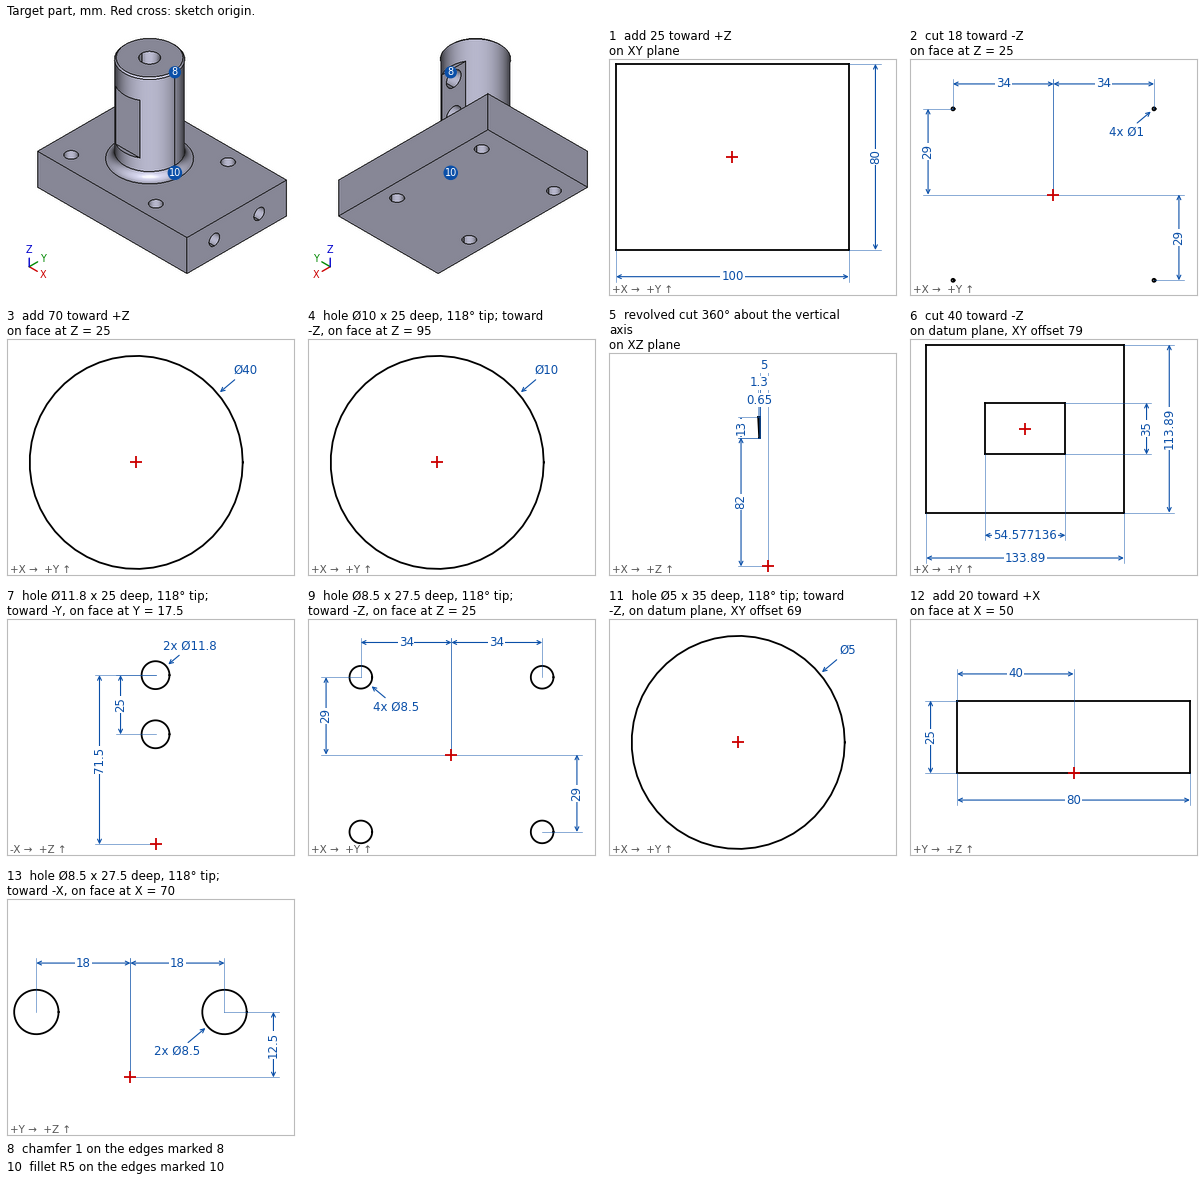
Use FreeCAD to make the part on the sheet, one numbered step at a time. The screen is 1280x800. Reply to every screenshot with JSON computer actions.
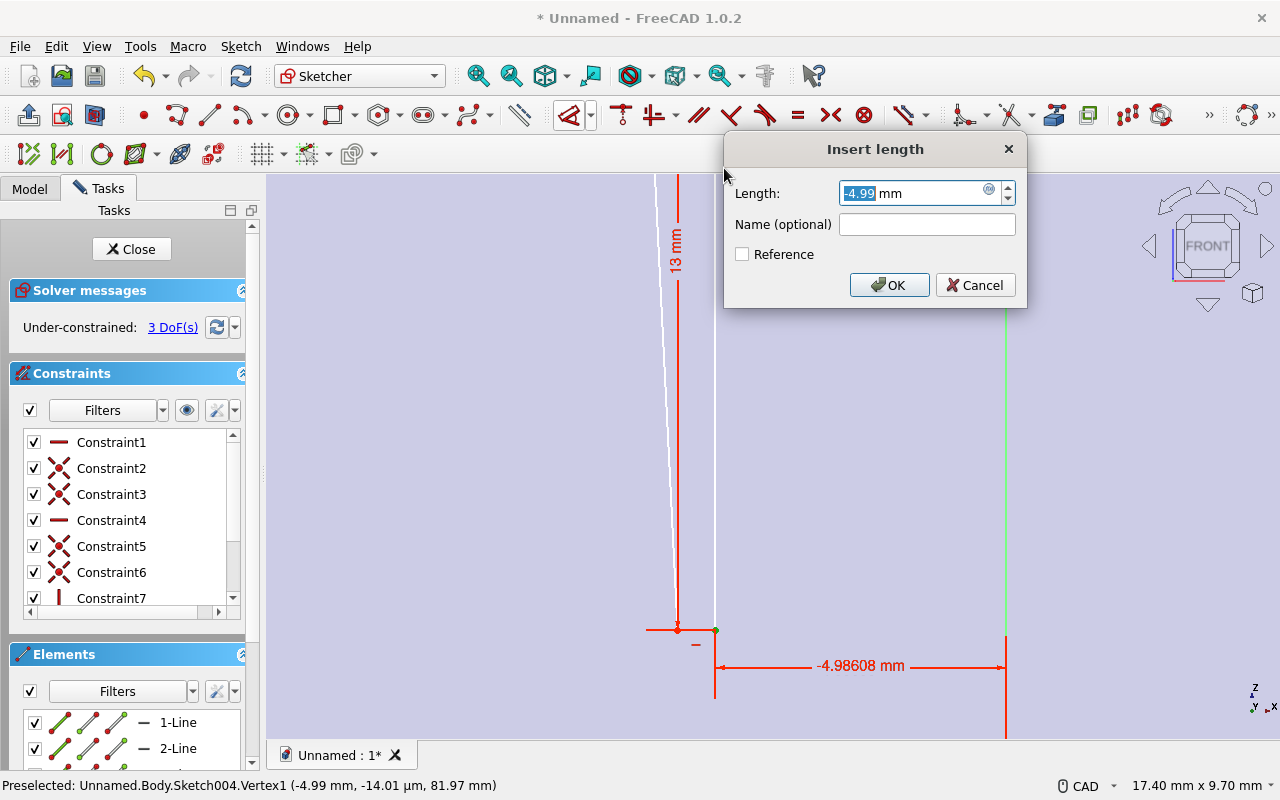
{"action": "type", "text": "-5"}
{"action": "key", "text": "Return"}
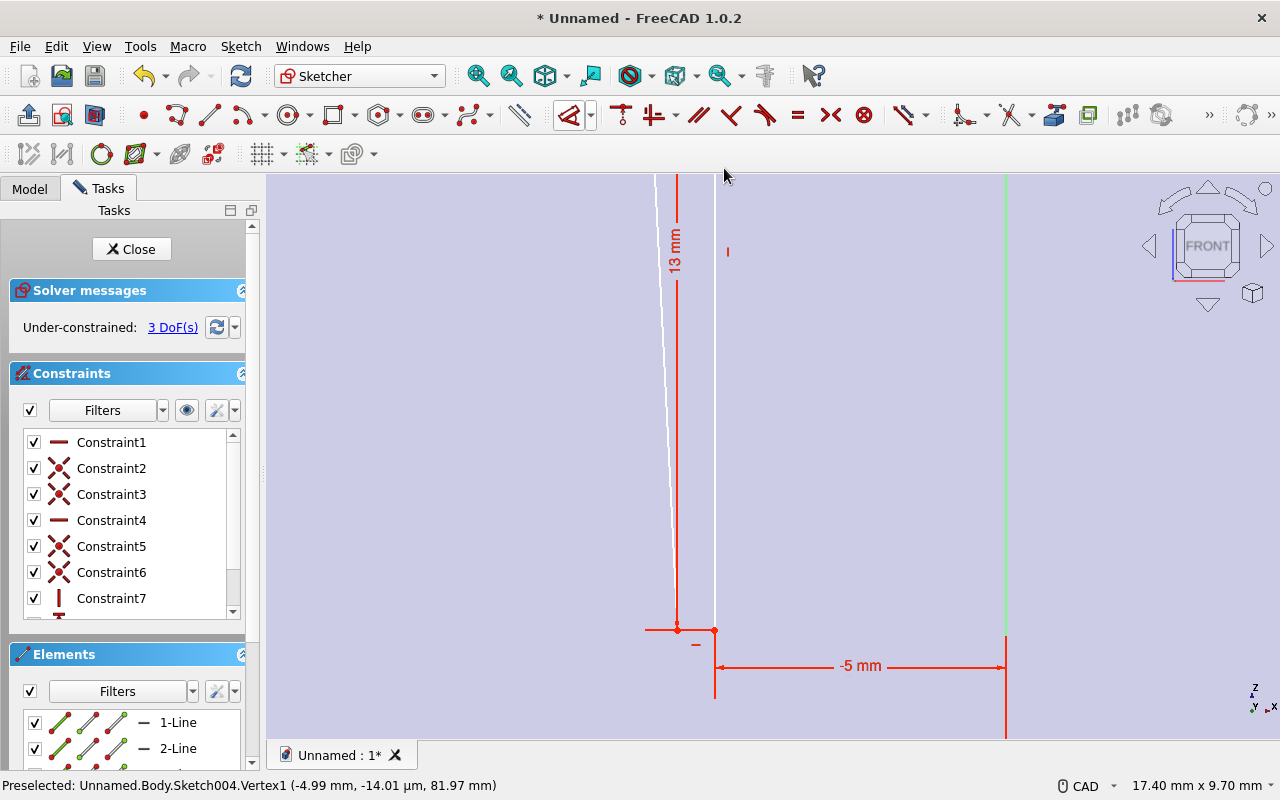
{"action": "scroll", "coordinate": [727, 626], "scroll_direction": "down", "scroll_amount": 4}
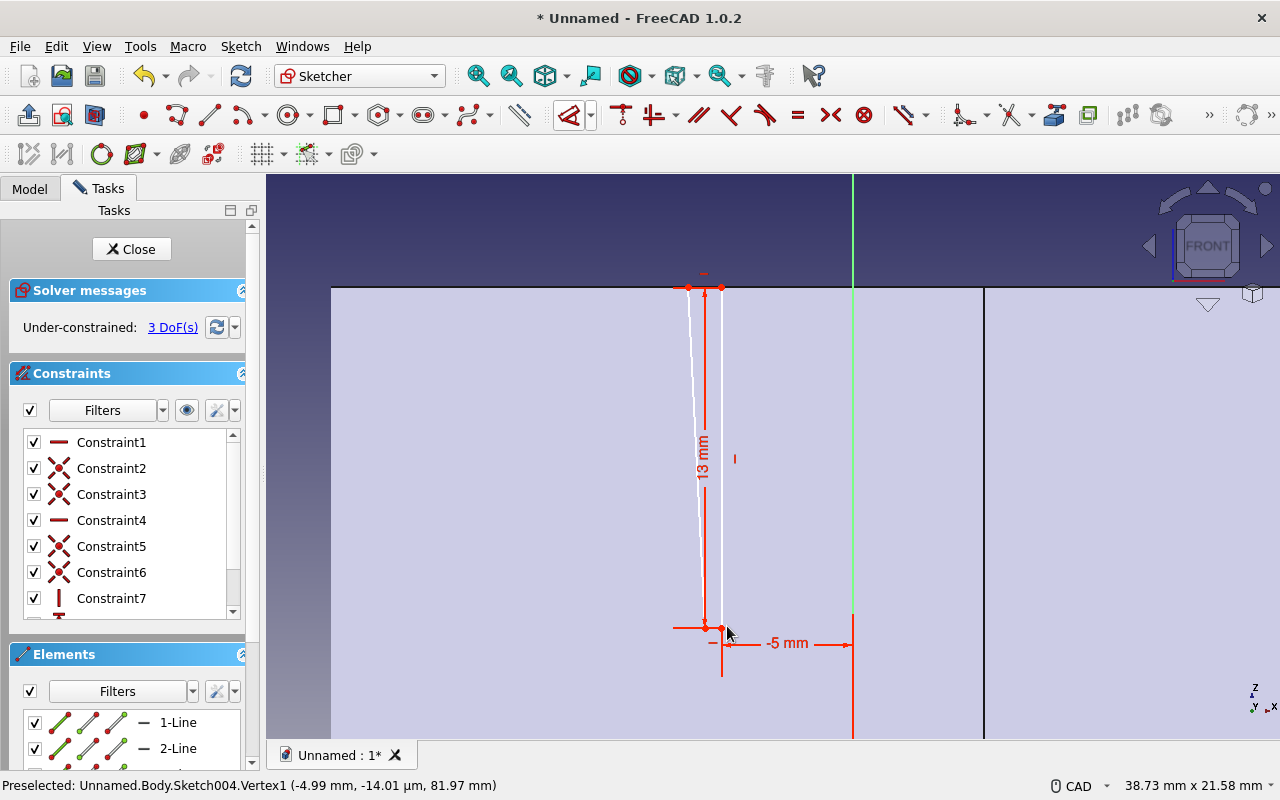
{"action": "scroll", "coordinate": [698, 288], "scroll_direction": "up", "scroll_amount": 2}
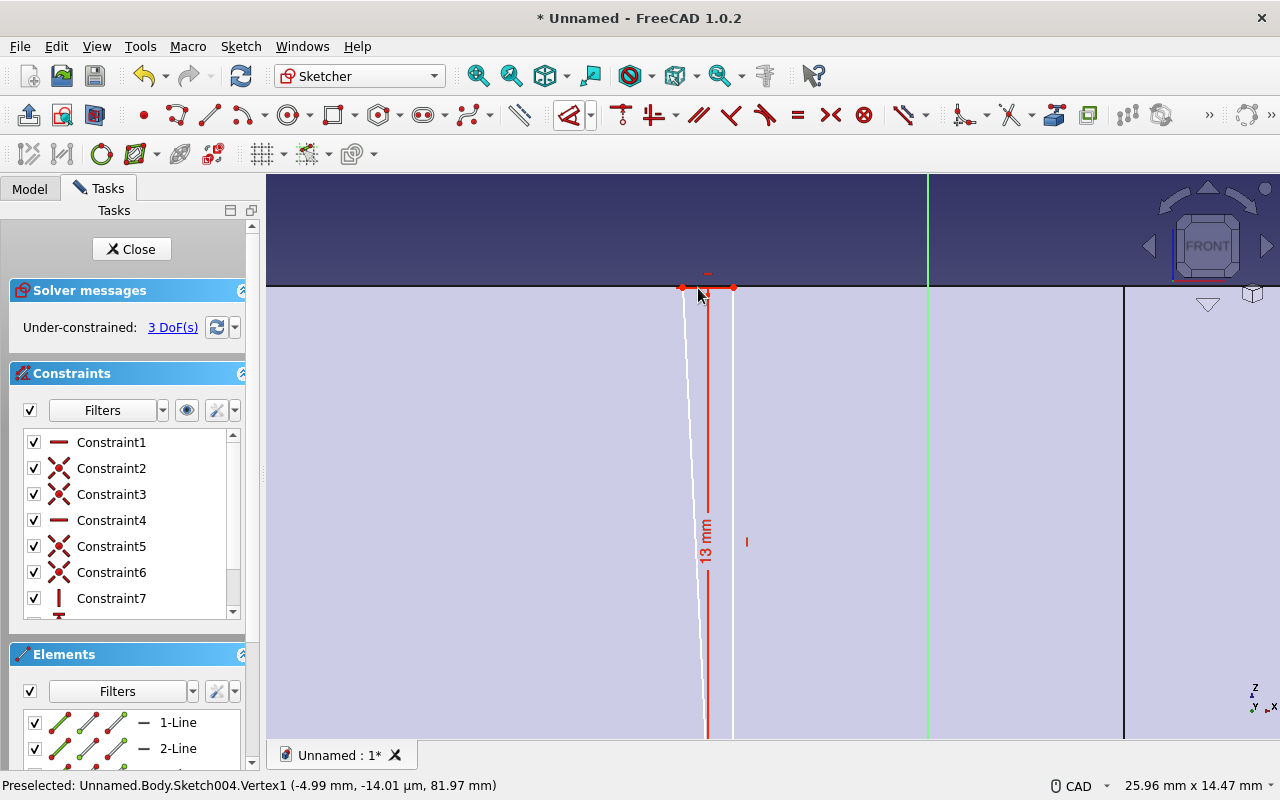
{"action": "left_click", "coordinate": [698, 288]}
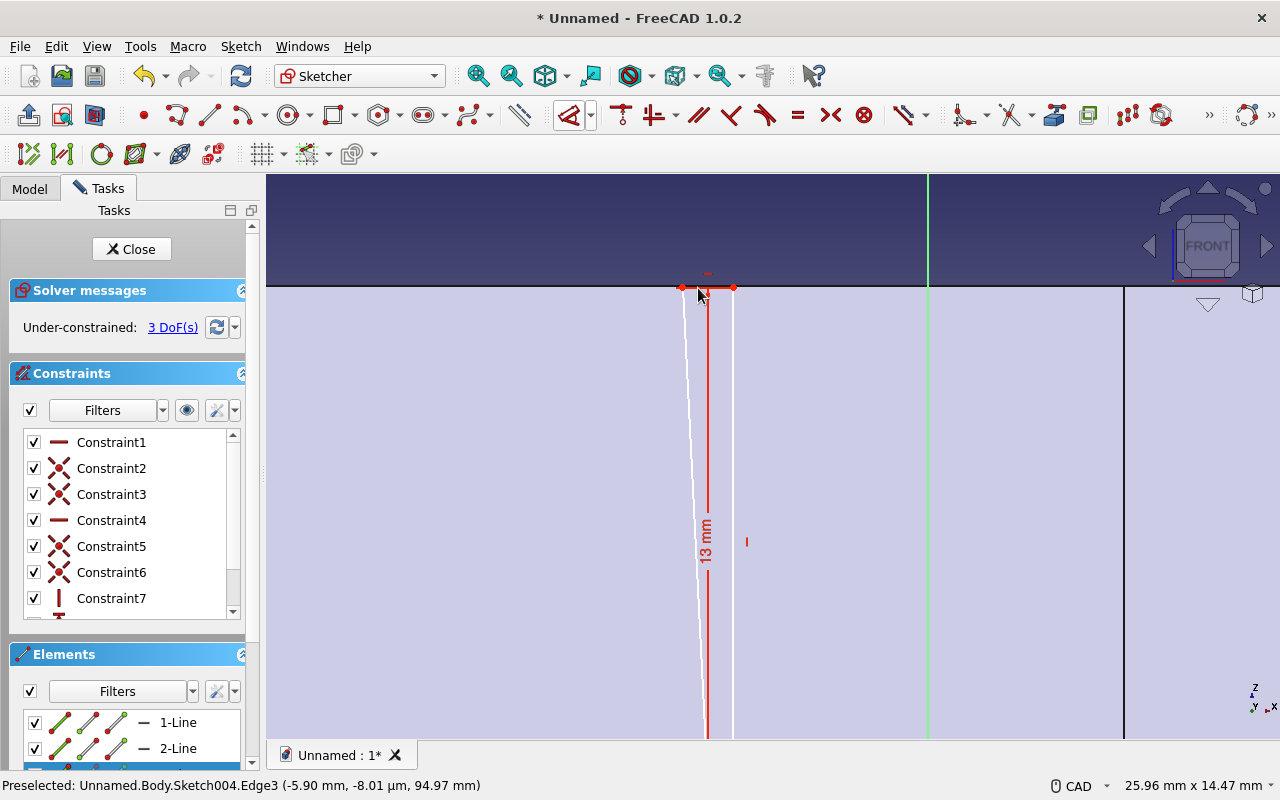
{"action": "left_click", "coordinate": [590, 116]}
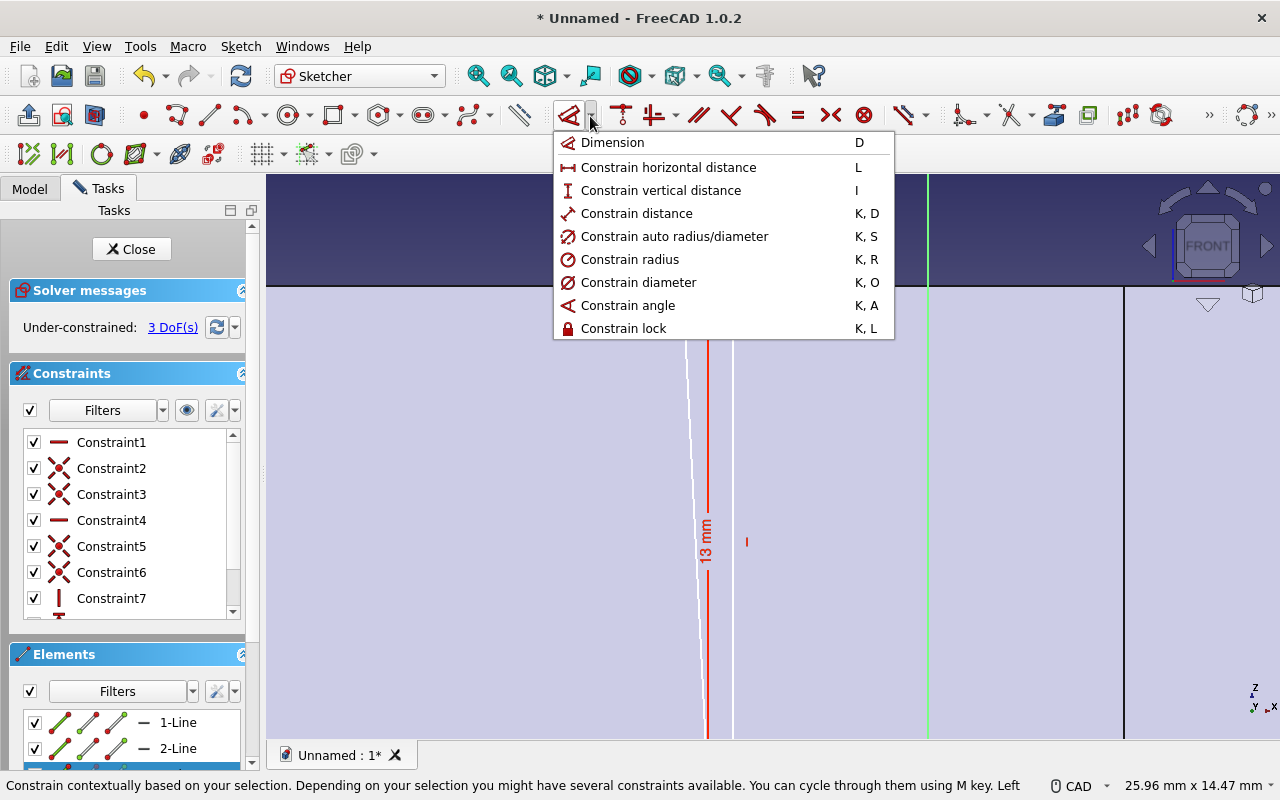
{"action": "left_click", "coordinate": [724, 168]}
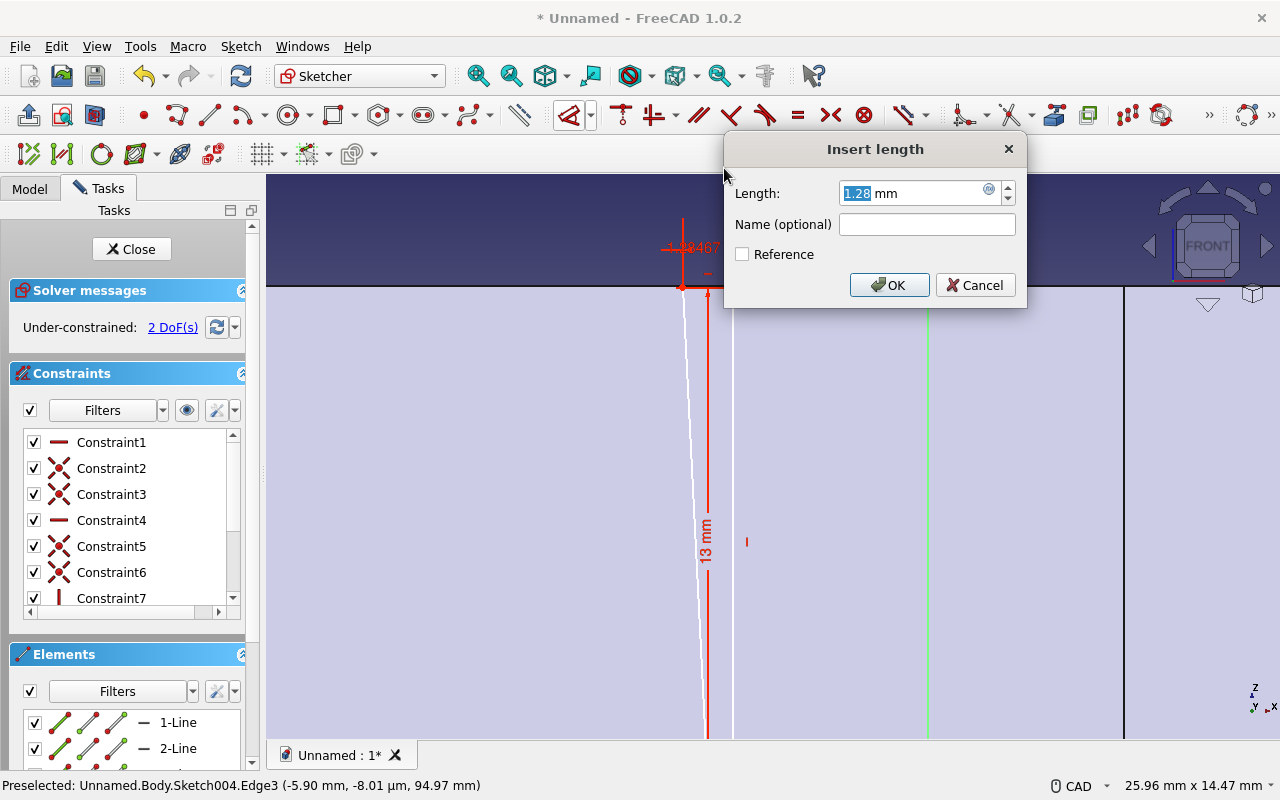
{"action": "type", "text": "1.3"}
{"action": "key", "text": "Return"}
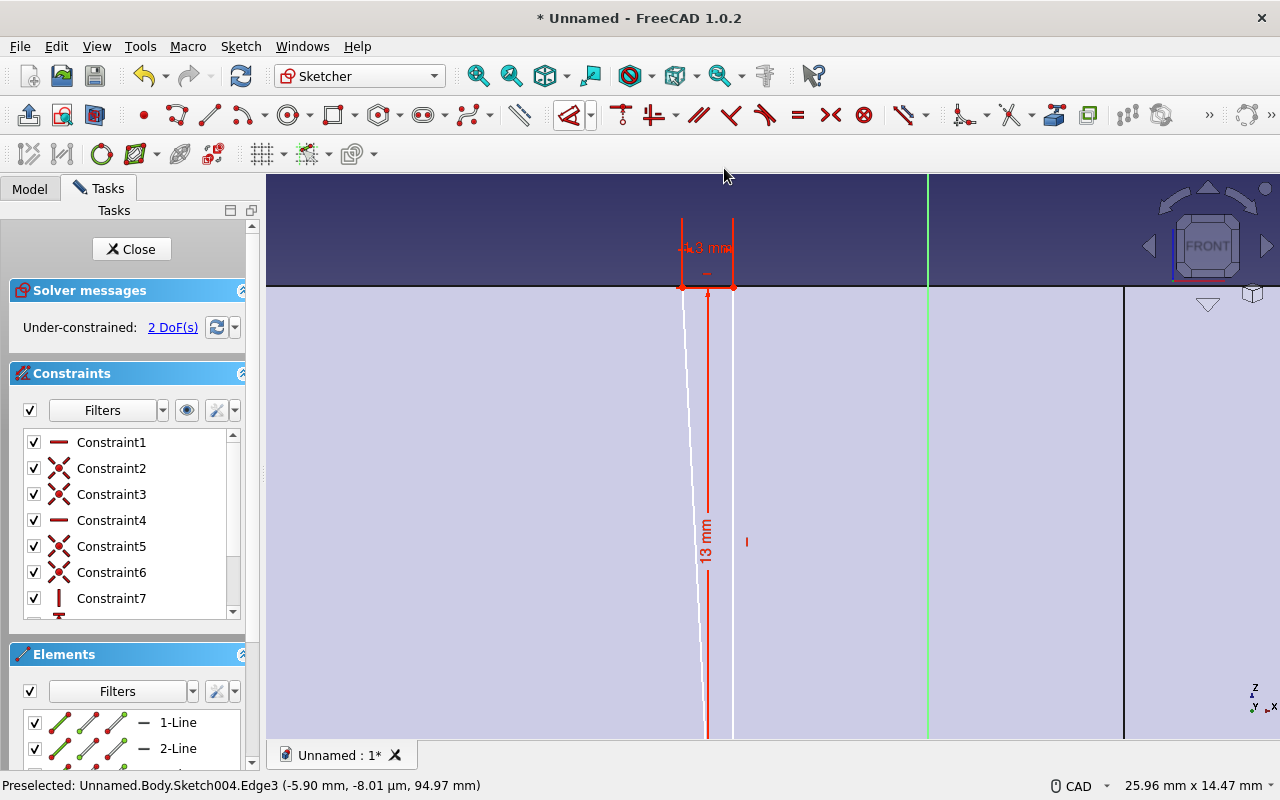
{"action": "scroll", "coordinate": [698, 286], "scroll_direction": "down", "scroll_amount": 2}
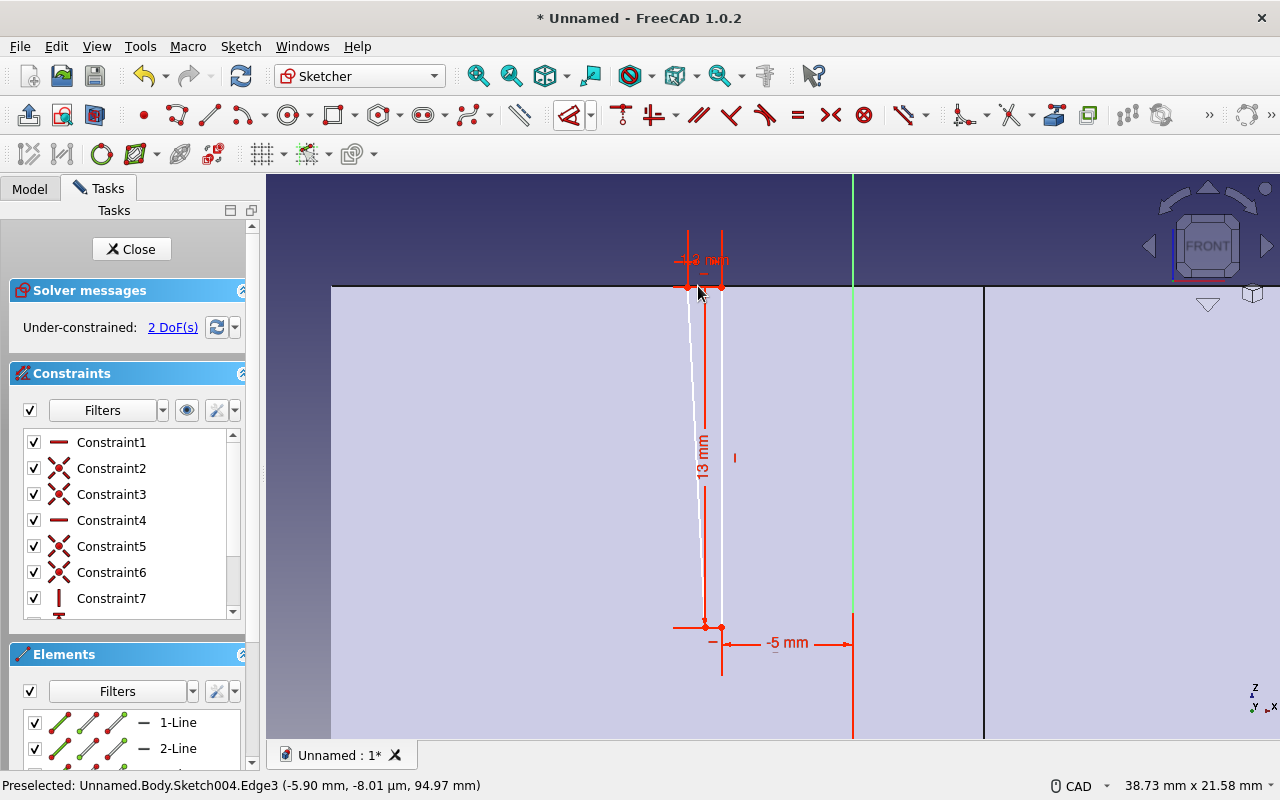
{"action": "left_click", "coordinate": [722, 628]}